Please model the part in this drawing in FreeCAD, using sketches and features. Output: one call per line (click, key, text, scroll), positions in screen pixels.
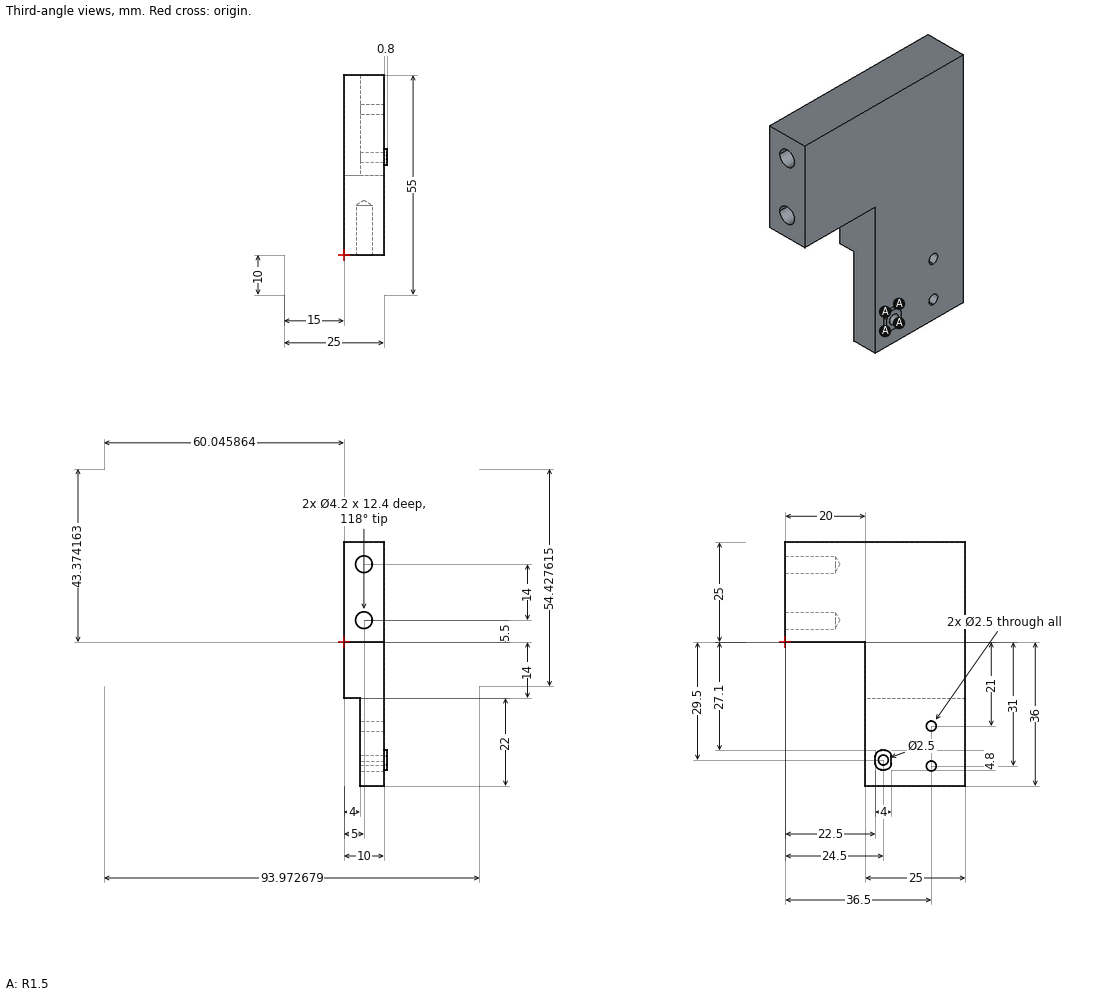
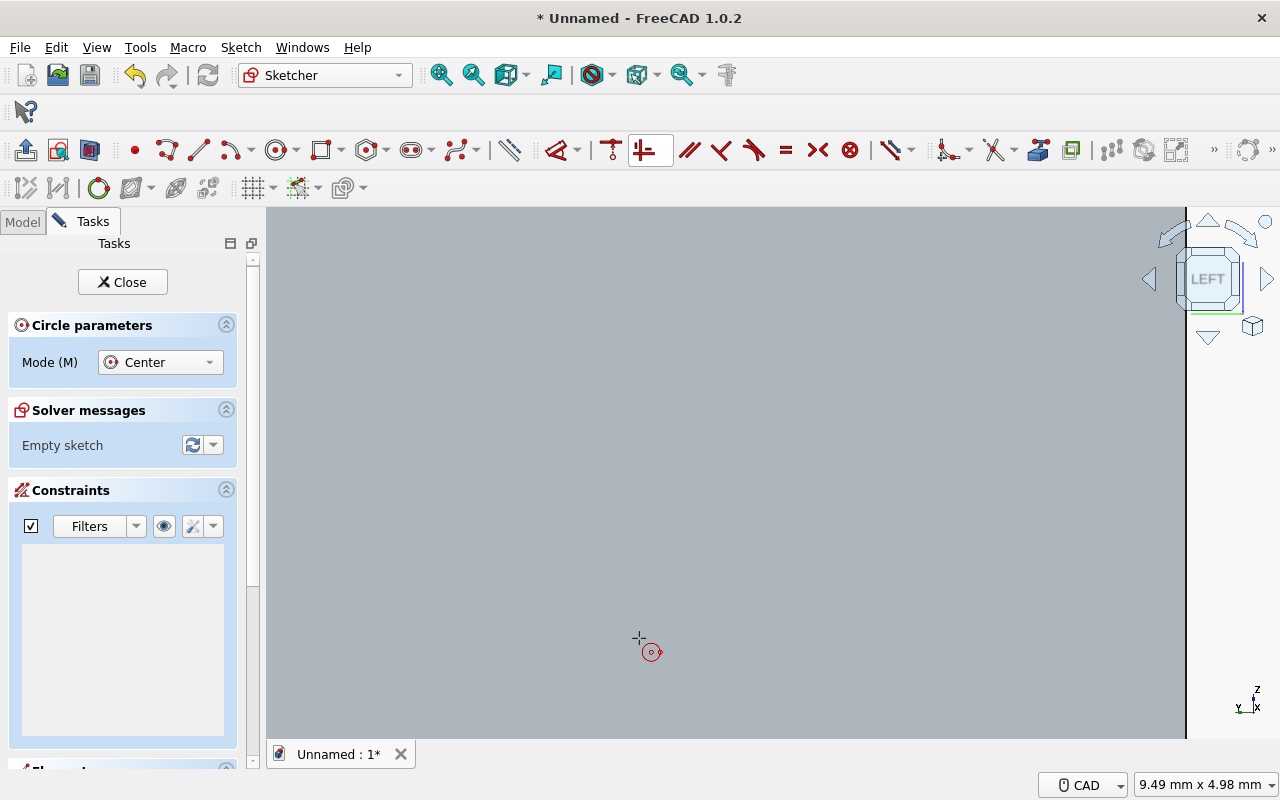
click(705, 461)
move(800, 366)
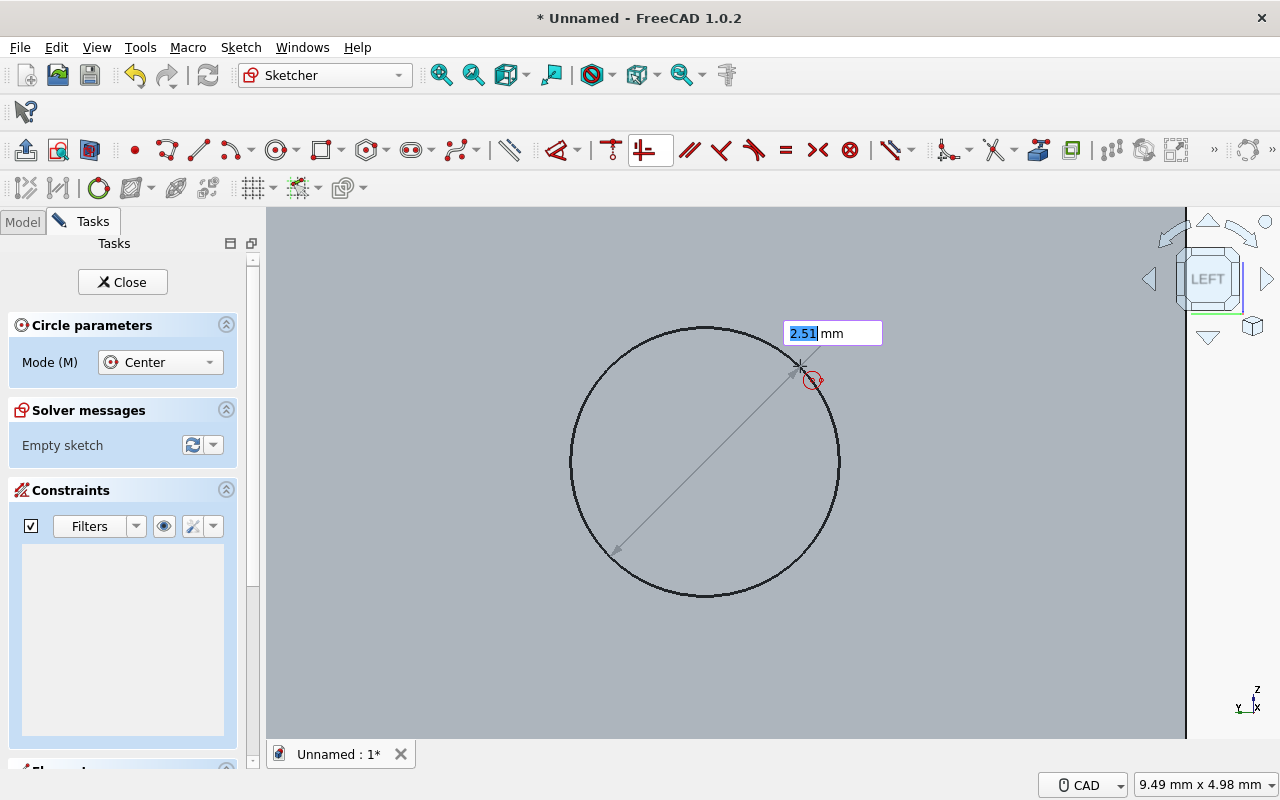
text(2.5)
key(Return)
key(Escape)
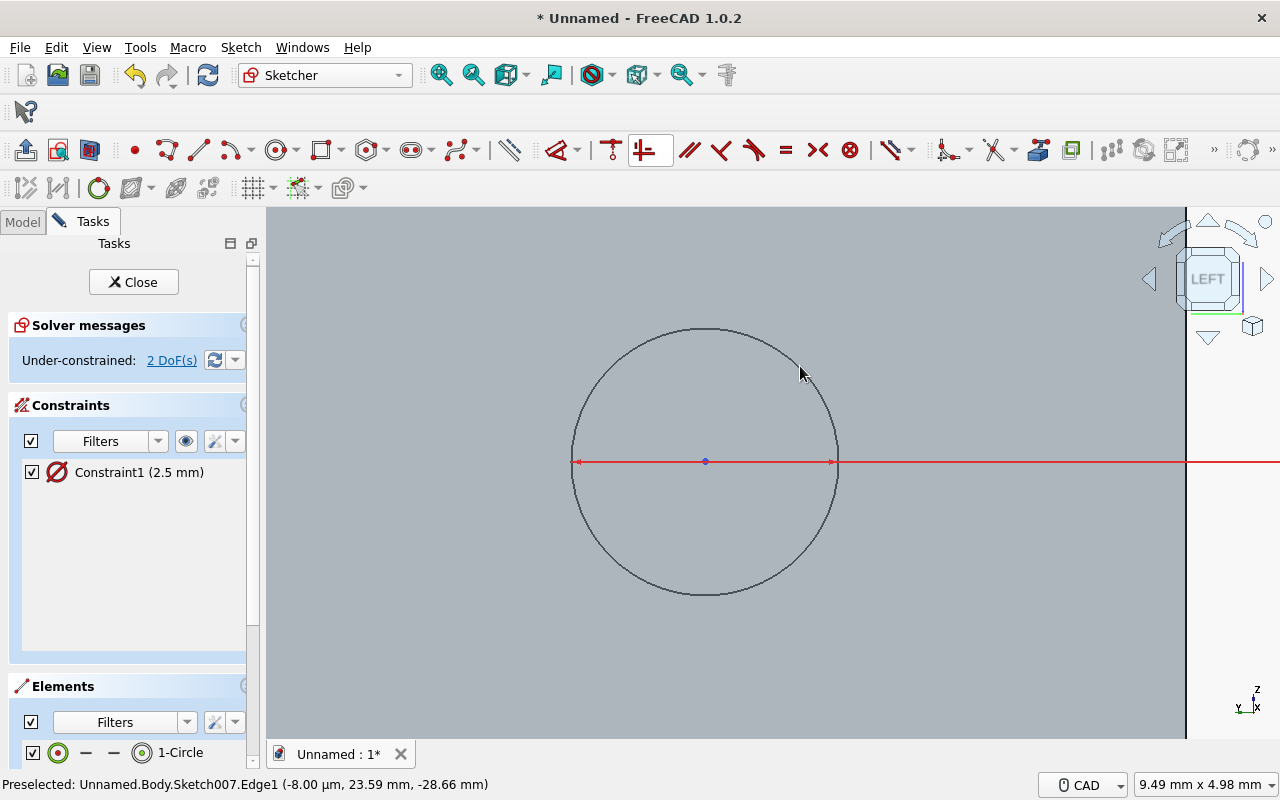
click(556, 150)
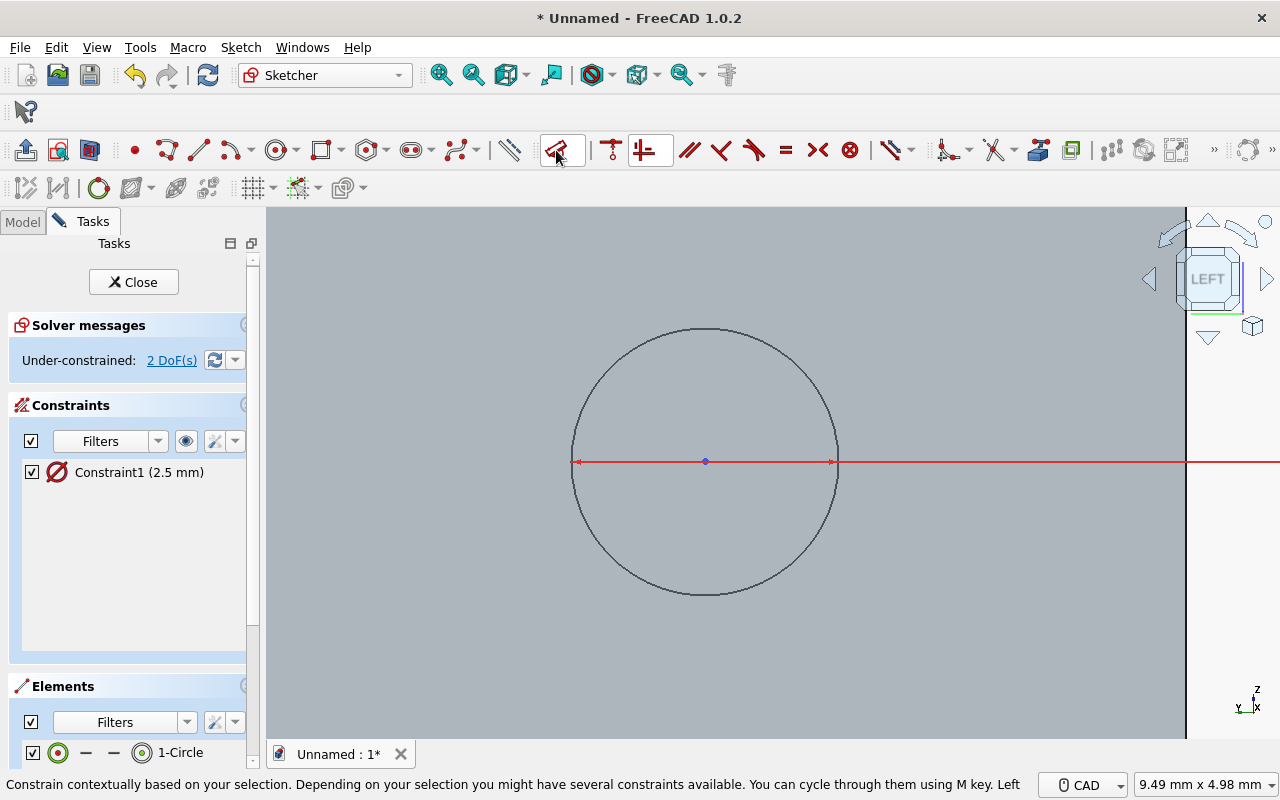
click(705, 462)
click(910, 496)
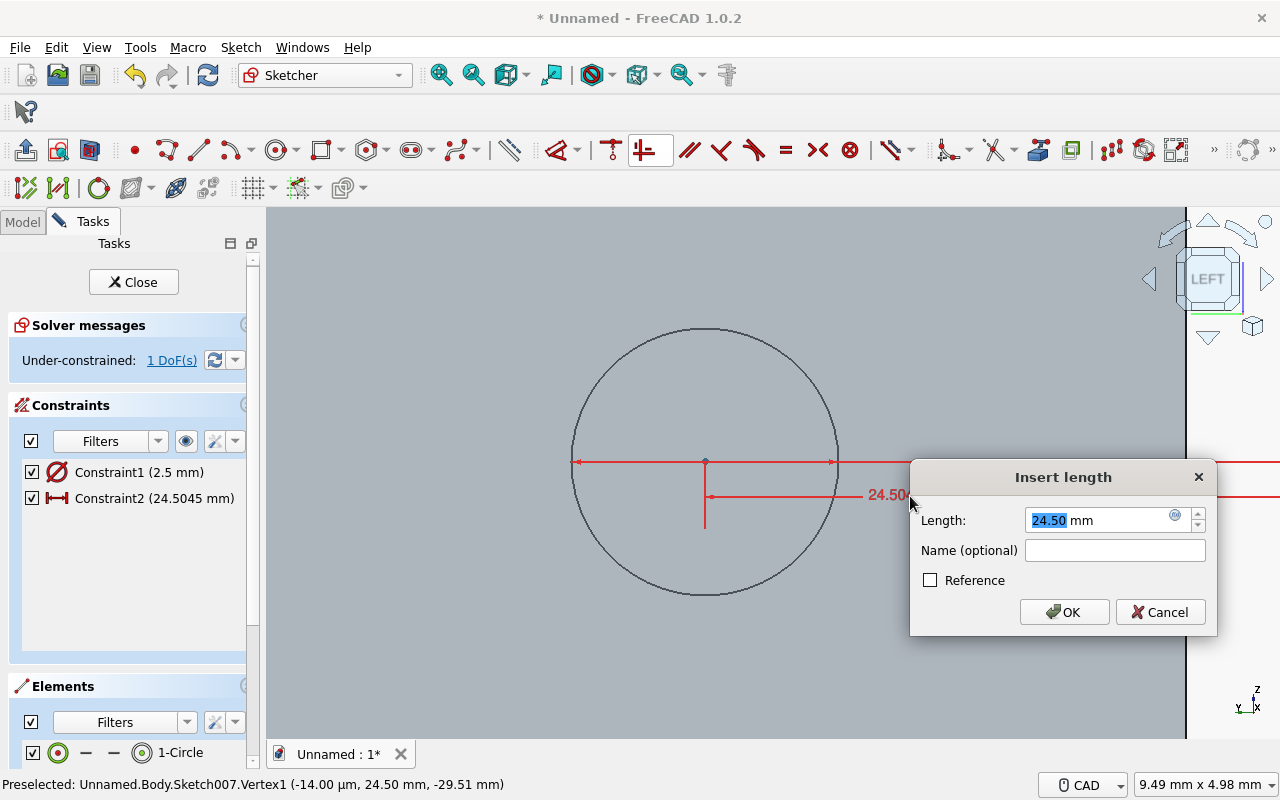
text(24.5)
key(Return)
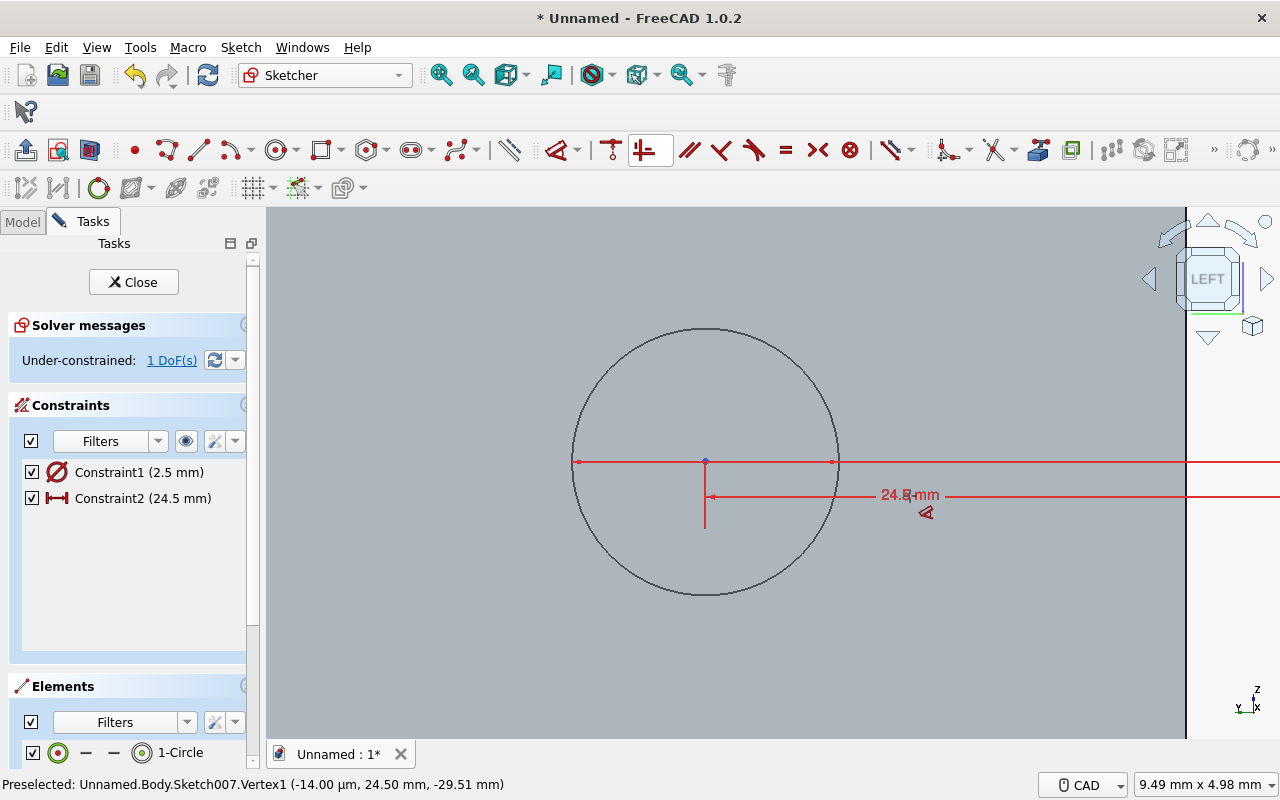
click(705, 462)
click(671, 348)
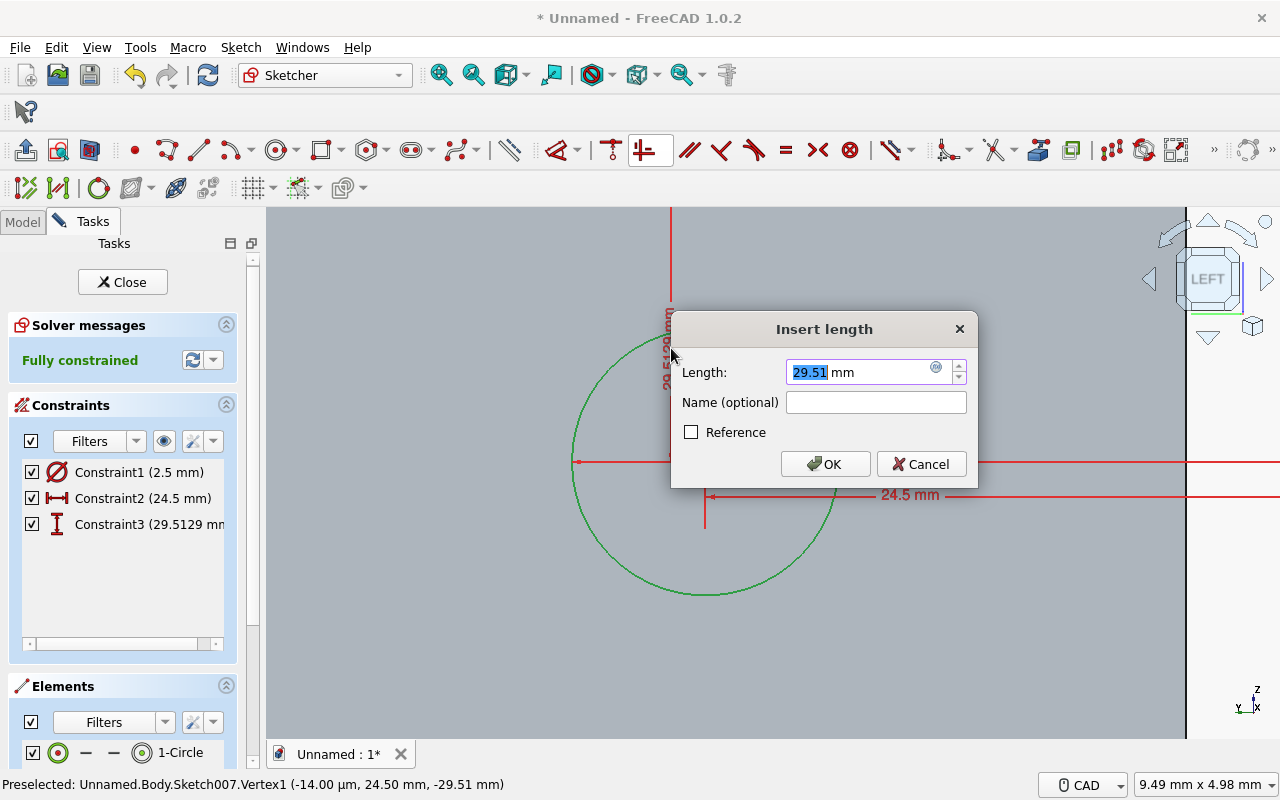
text(29.5)
key(Return)
key(Escape)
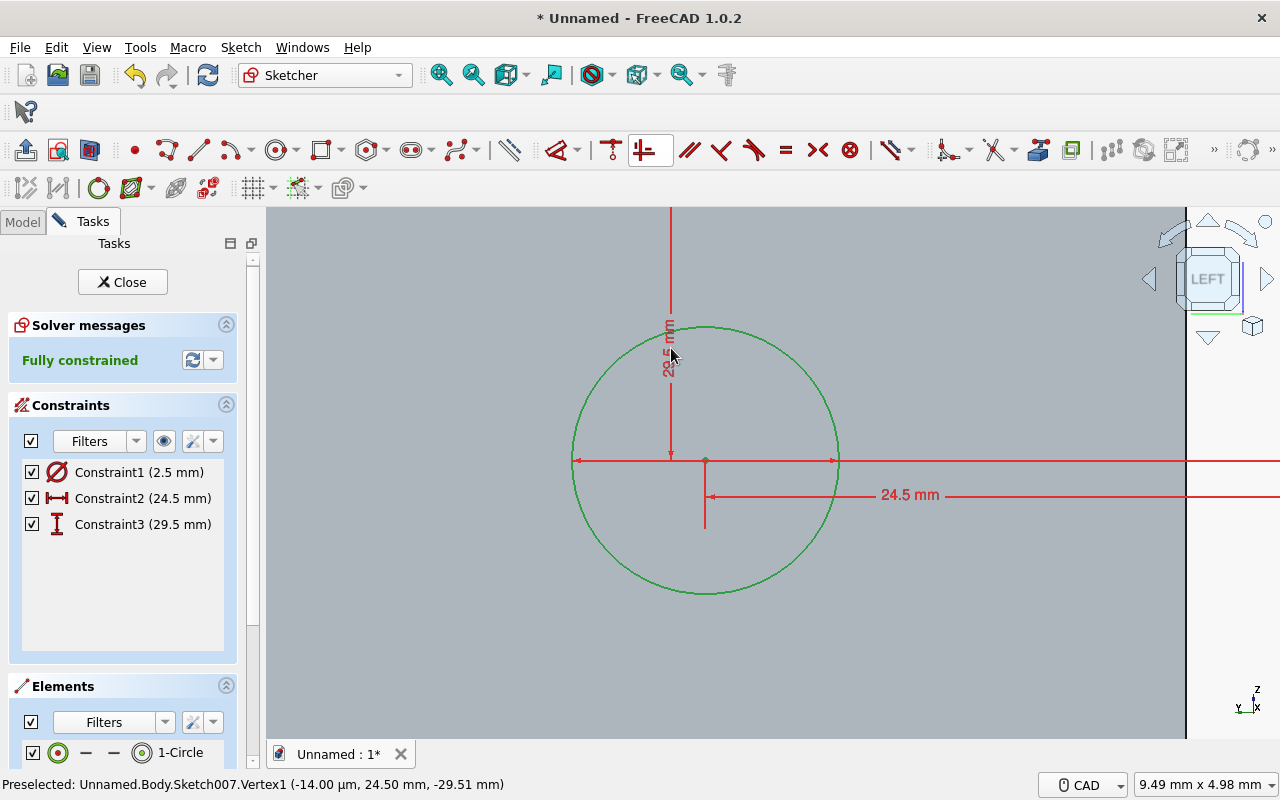
click(123, 282)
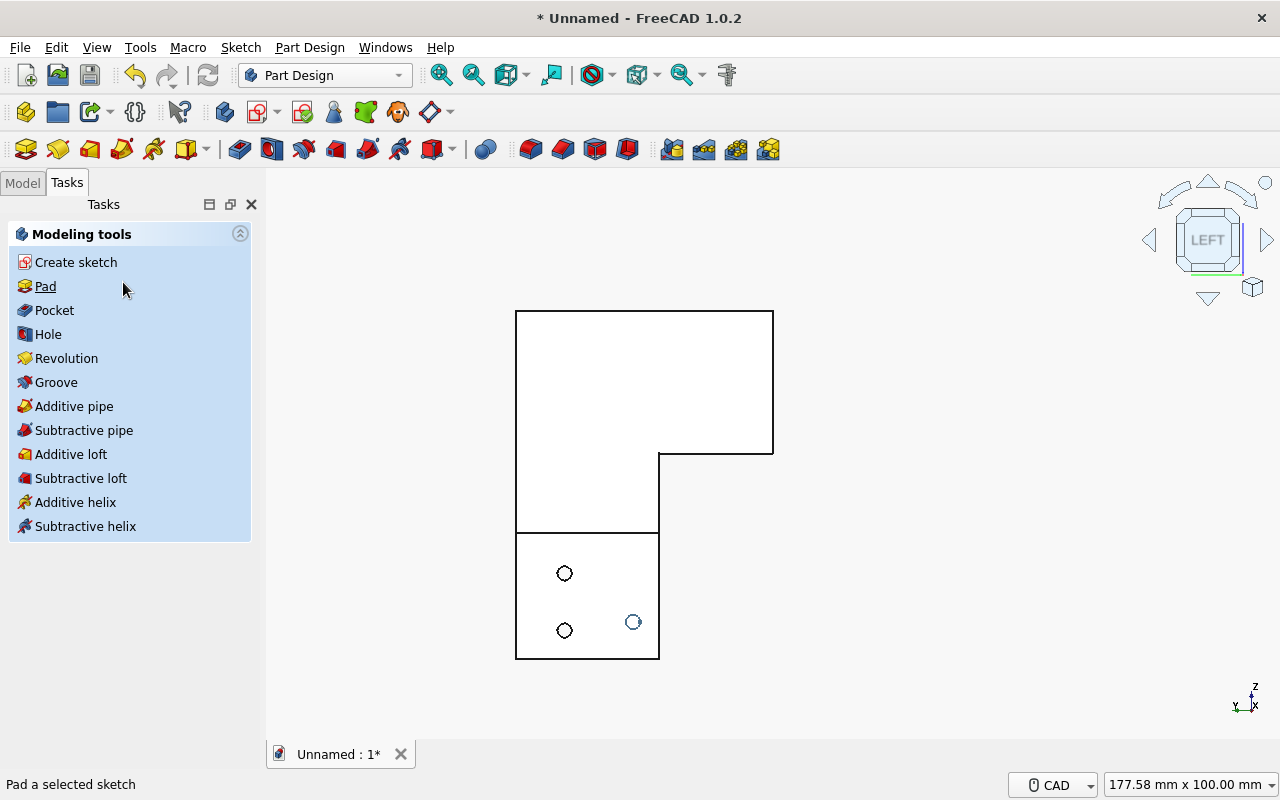
click(240, 150)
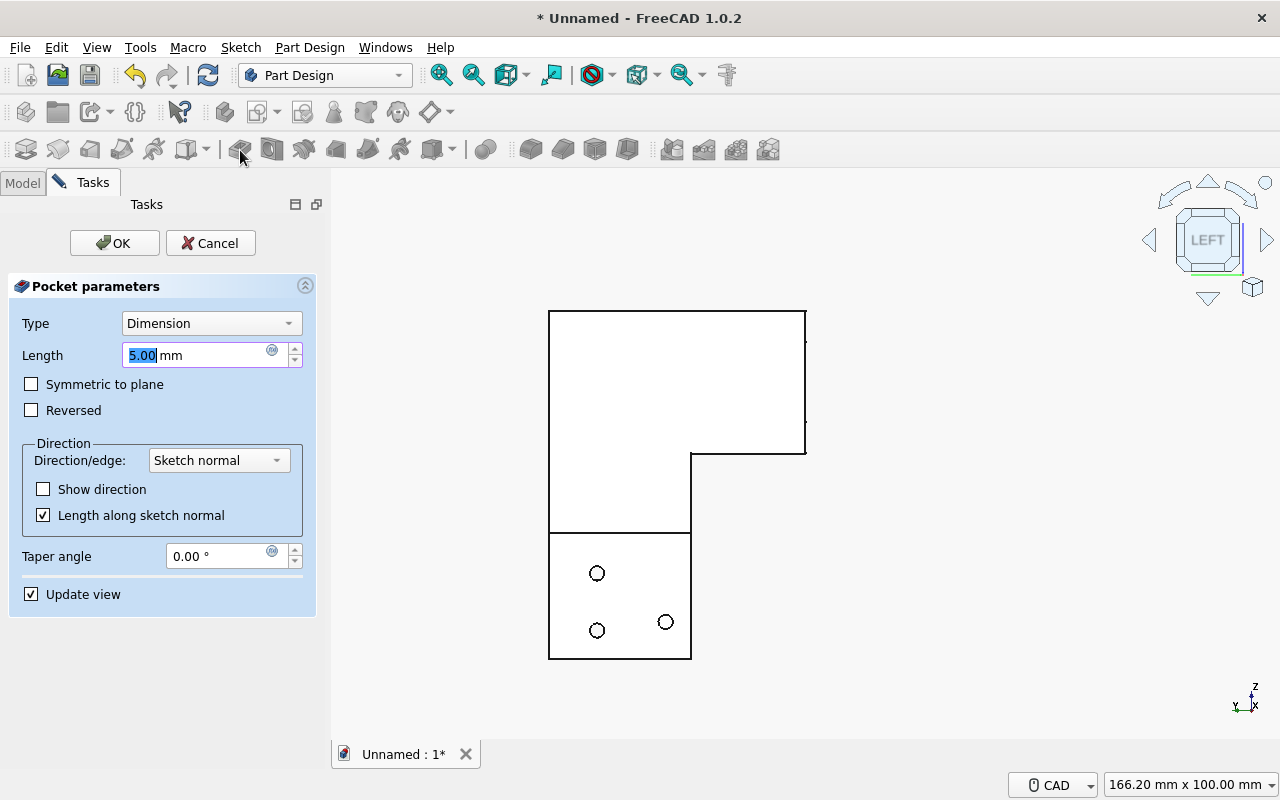
click(212, 324)